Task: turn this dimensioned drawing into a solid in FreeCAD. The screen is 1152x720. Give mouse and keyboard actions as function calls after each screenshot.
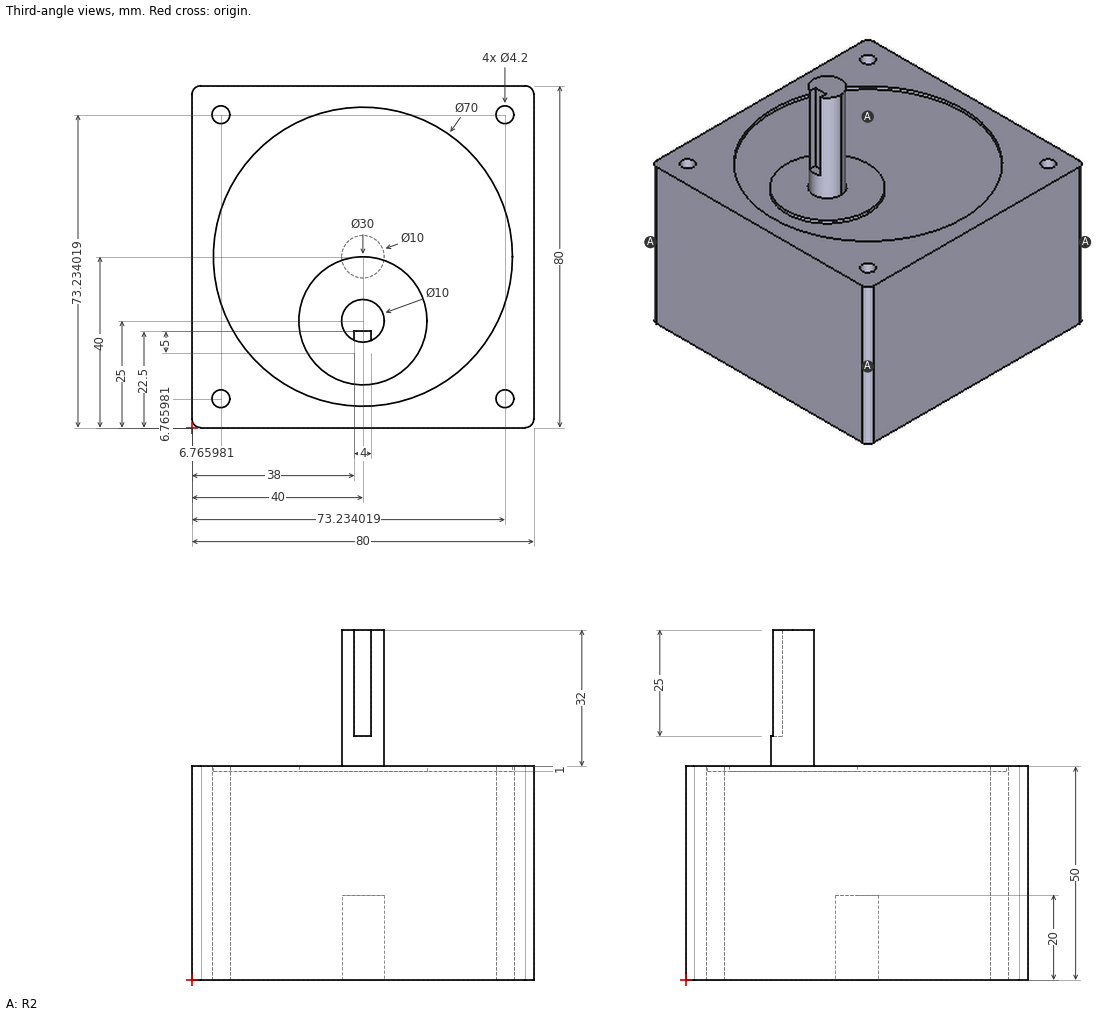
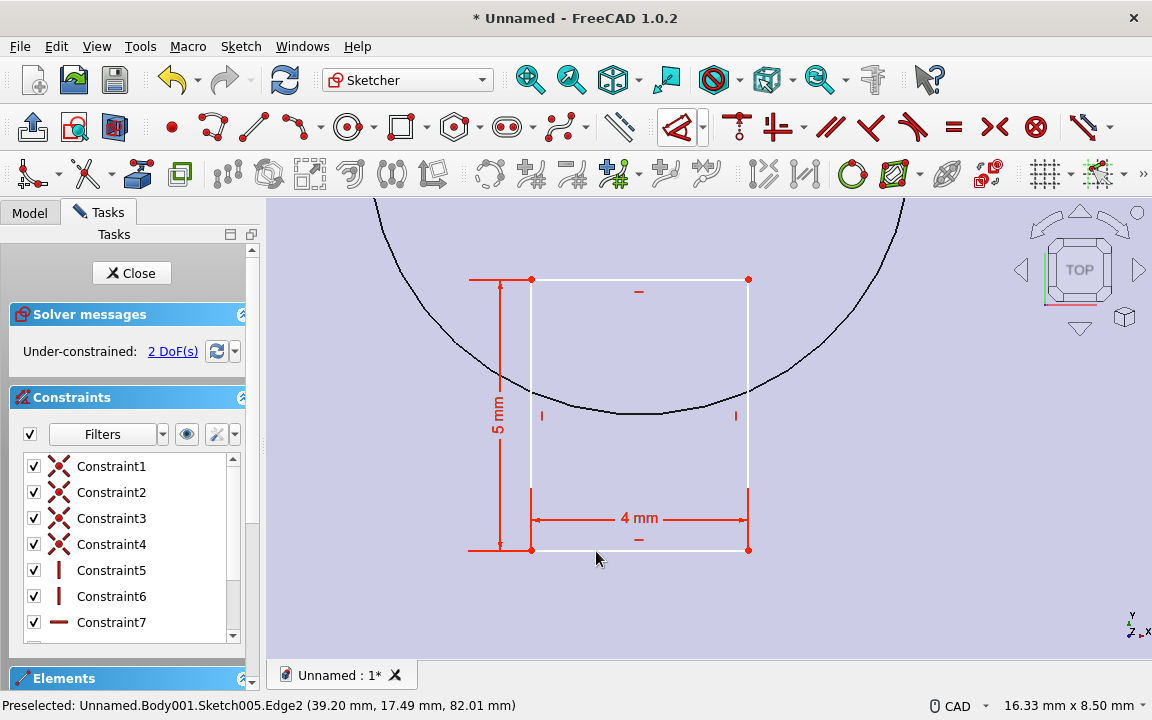
click(531, 280)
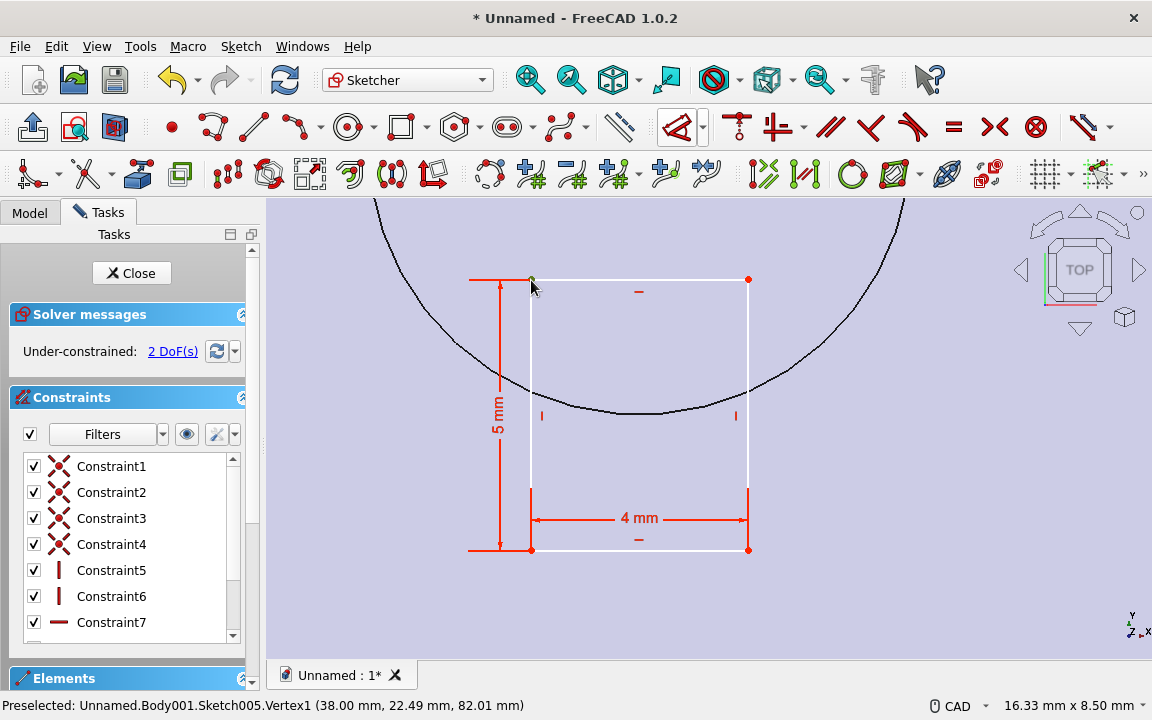
key(l)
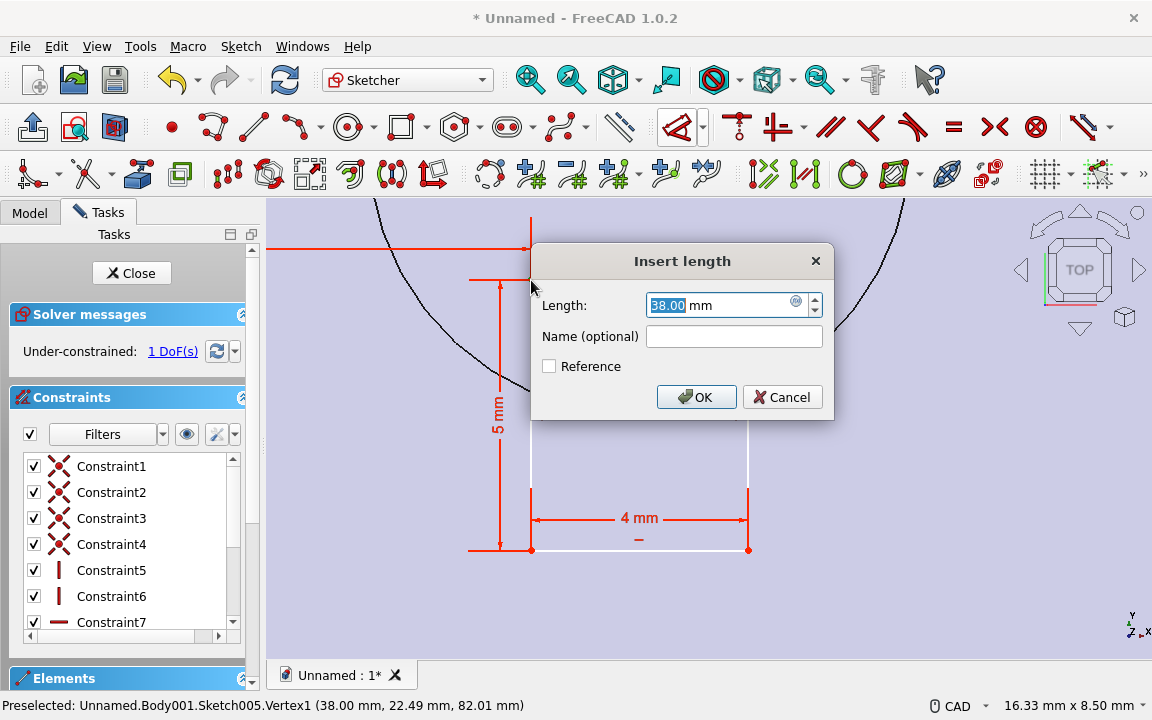
text(38)
key(Return)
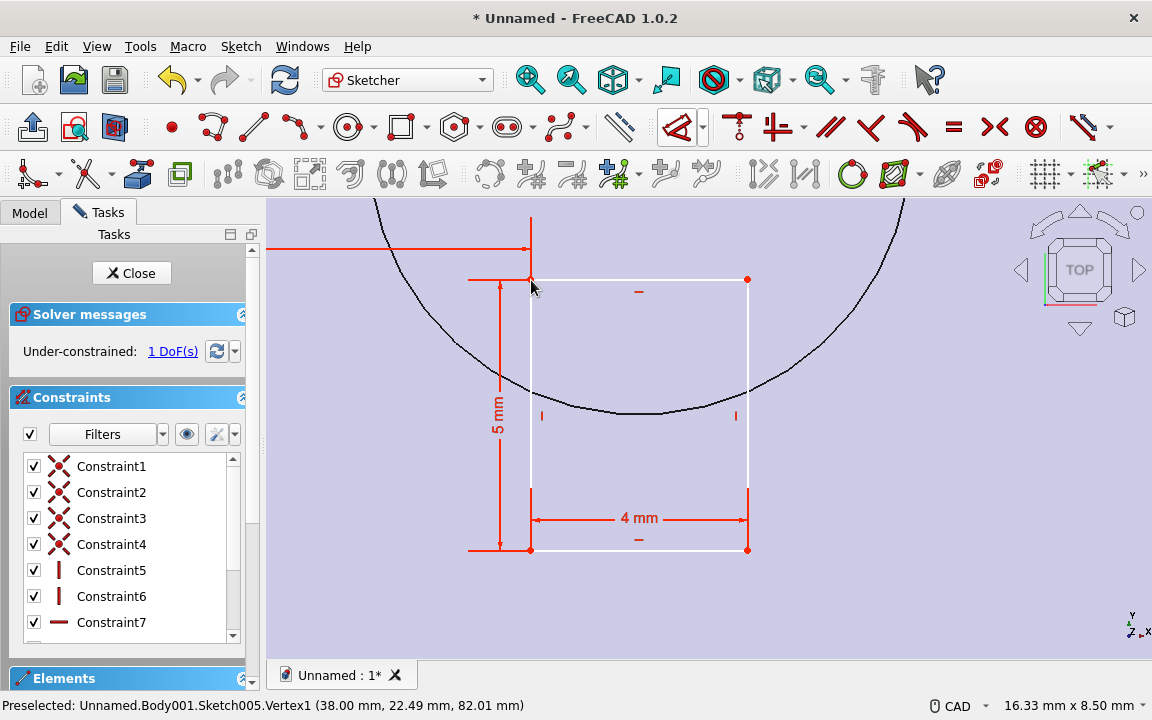
click(531, 280)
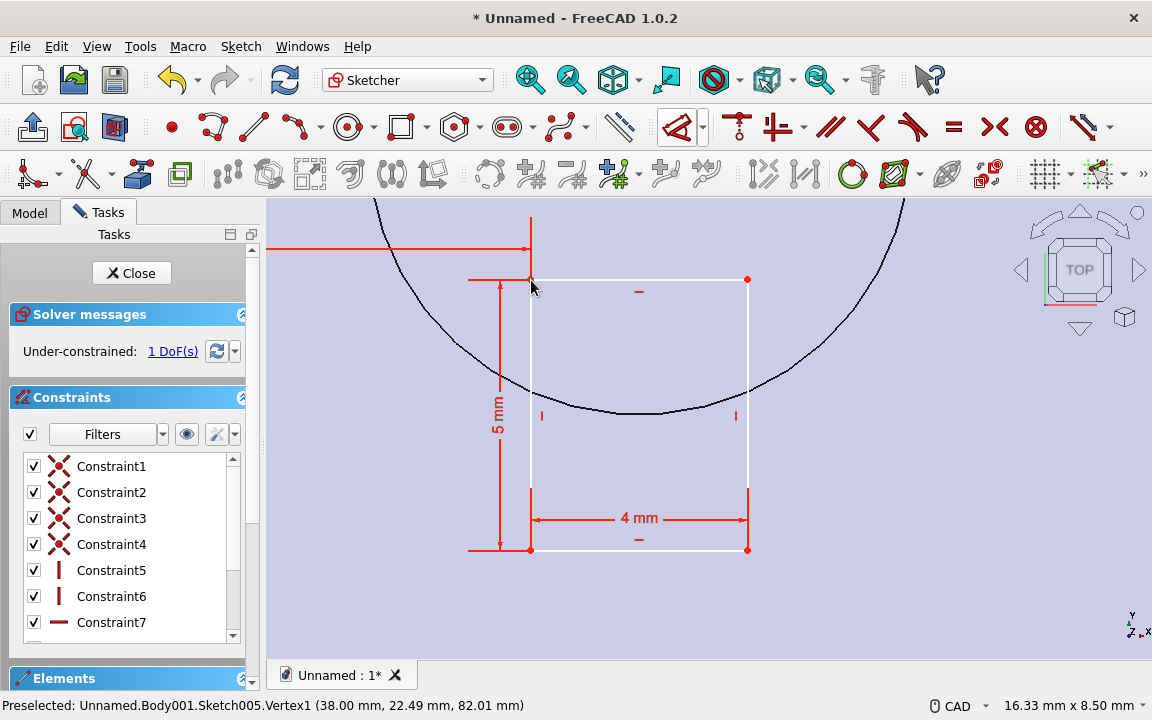
click(702, 128)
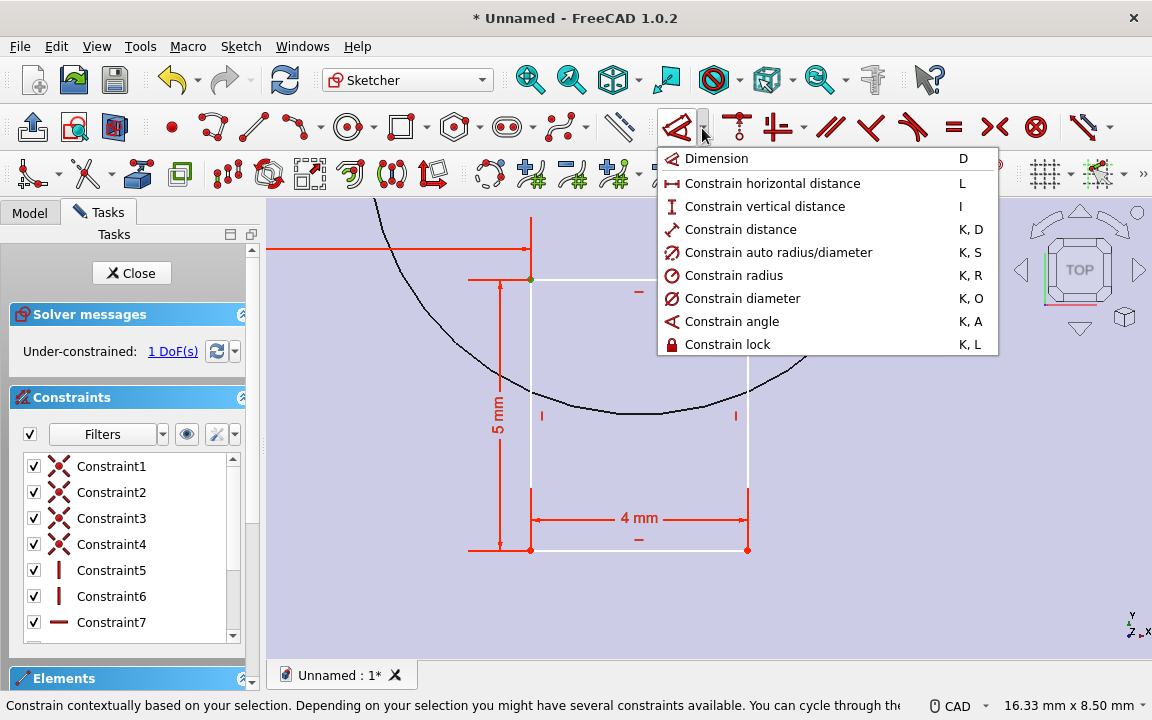
click(828, 206)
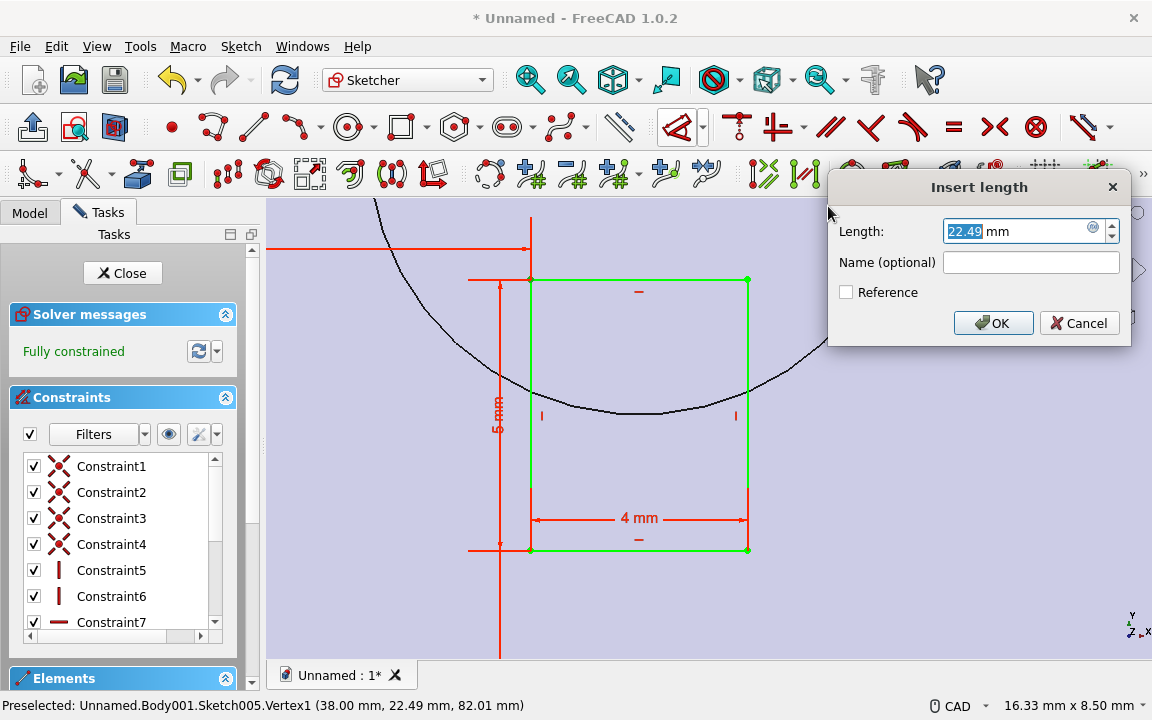
text(22.5)
key(Return)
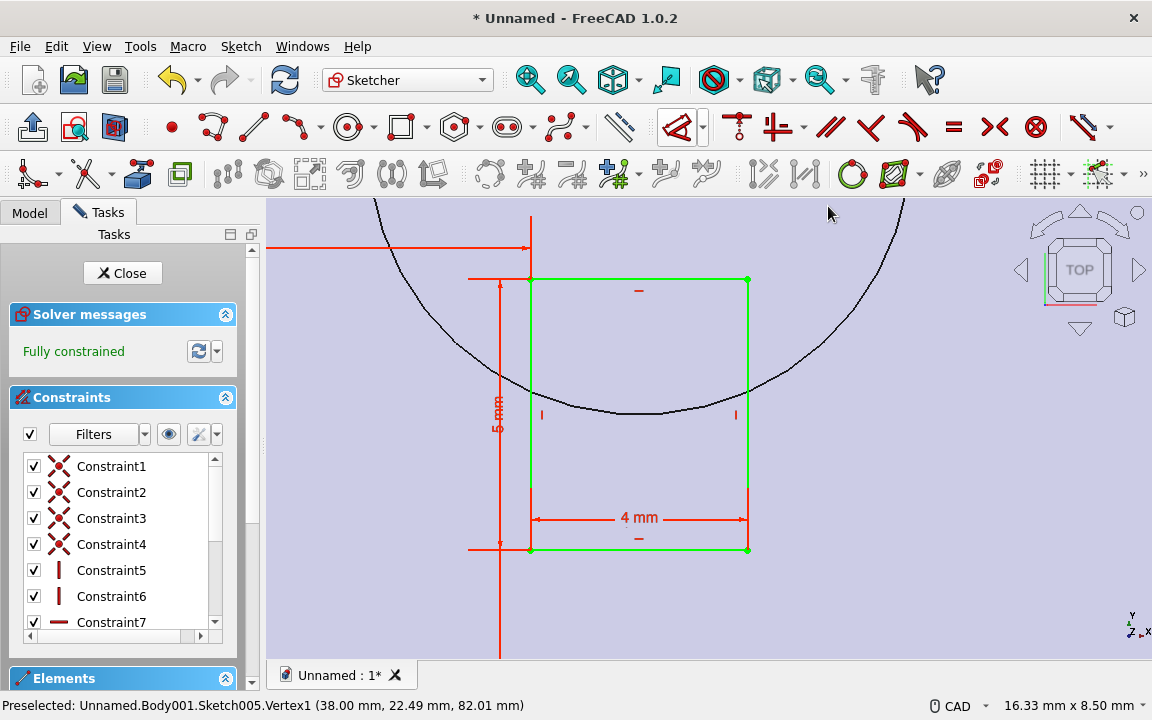
click(123, 273)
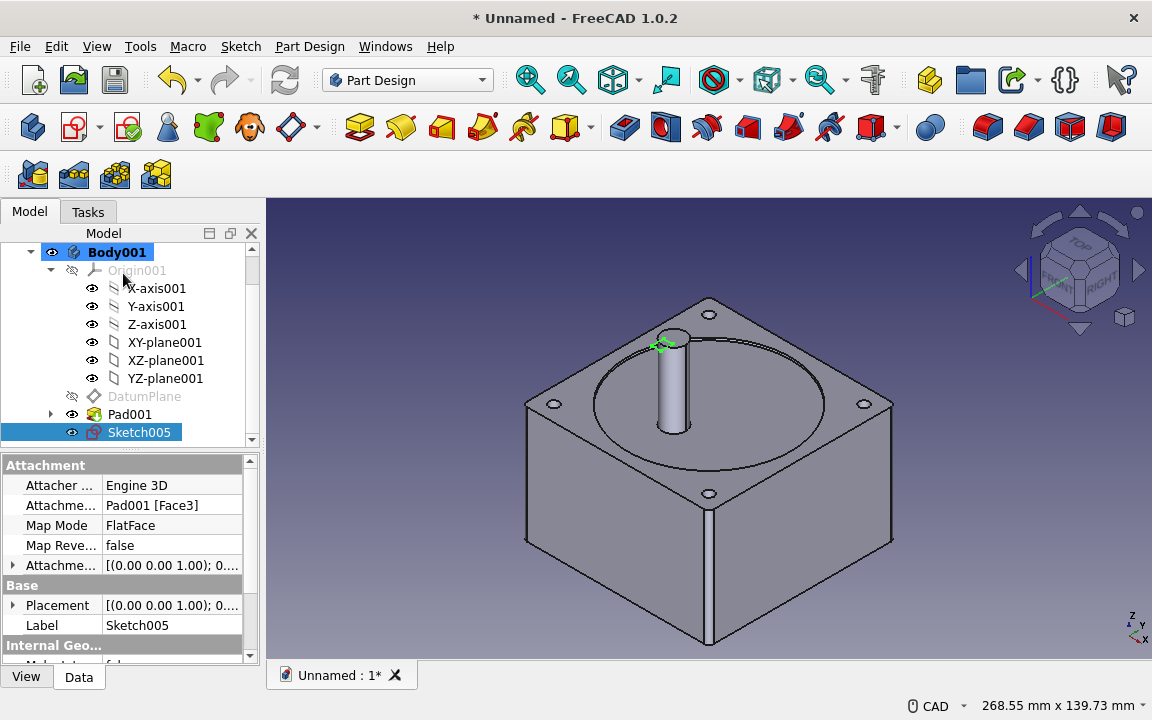
click(625, 128)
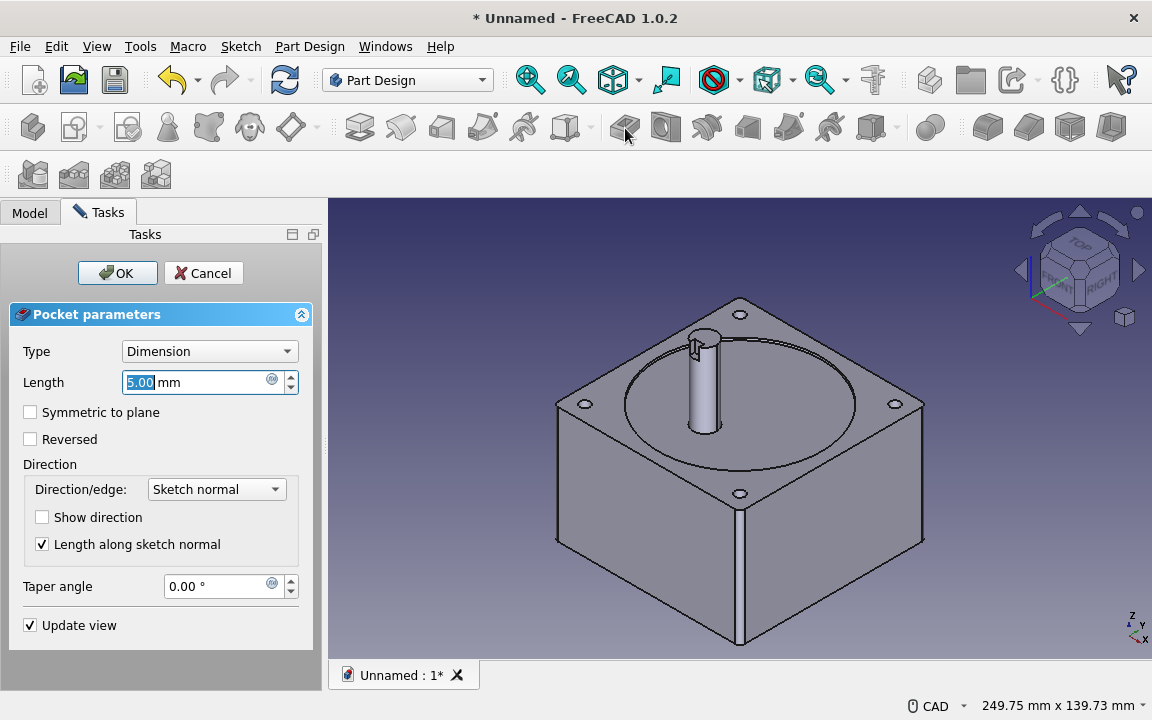
text(25)
key(Tab)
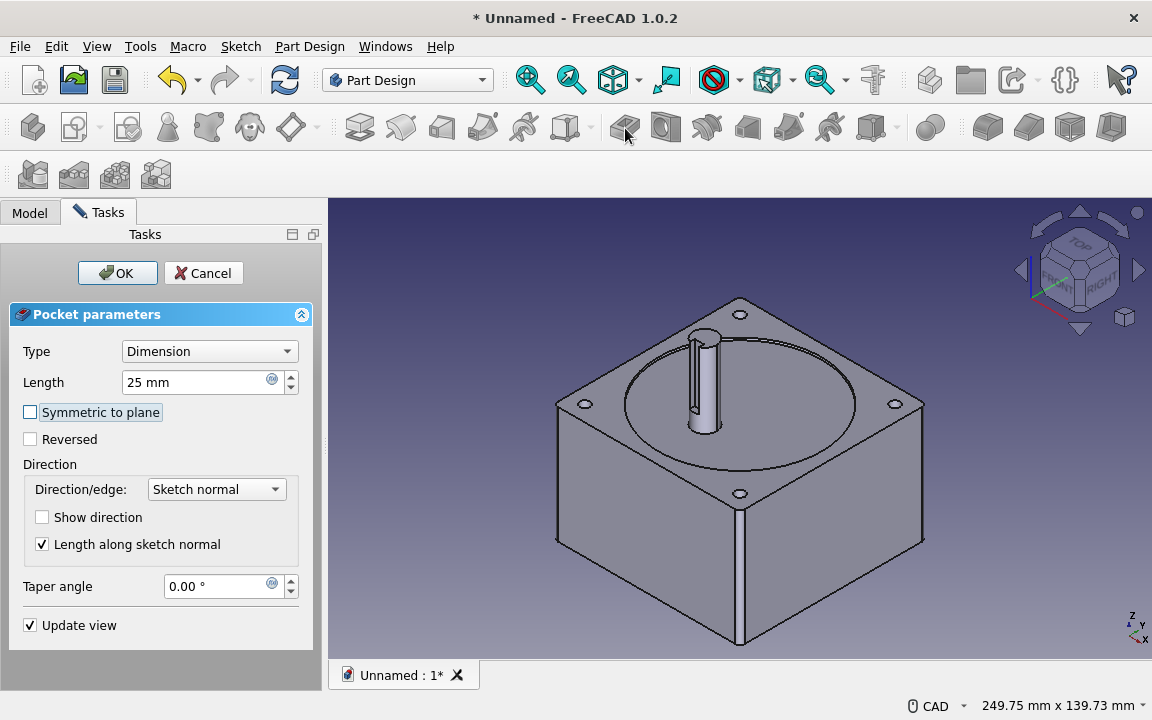
click(118, 273)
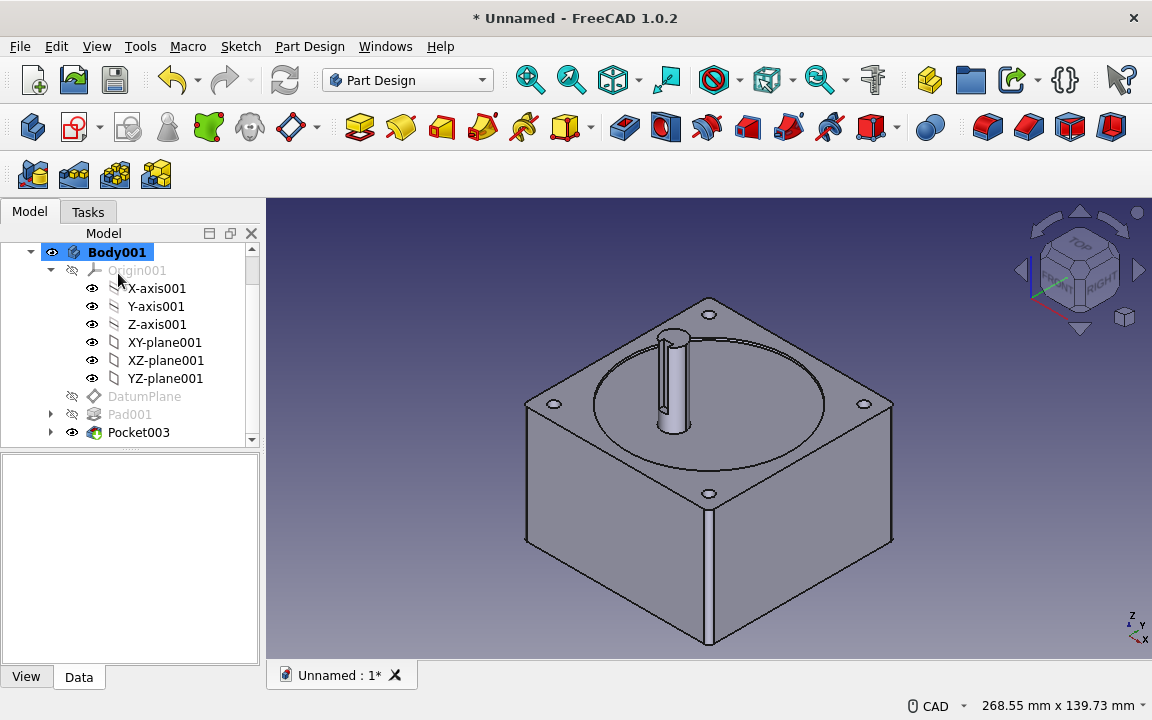
click(531, 80)